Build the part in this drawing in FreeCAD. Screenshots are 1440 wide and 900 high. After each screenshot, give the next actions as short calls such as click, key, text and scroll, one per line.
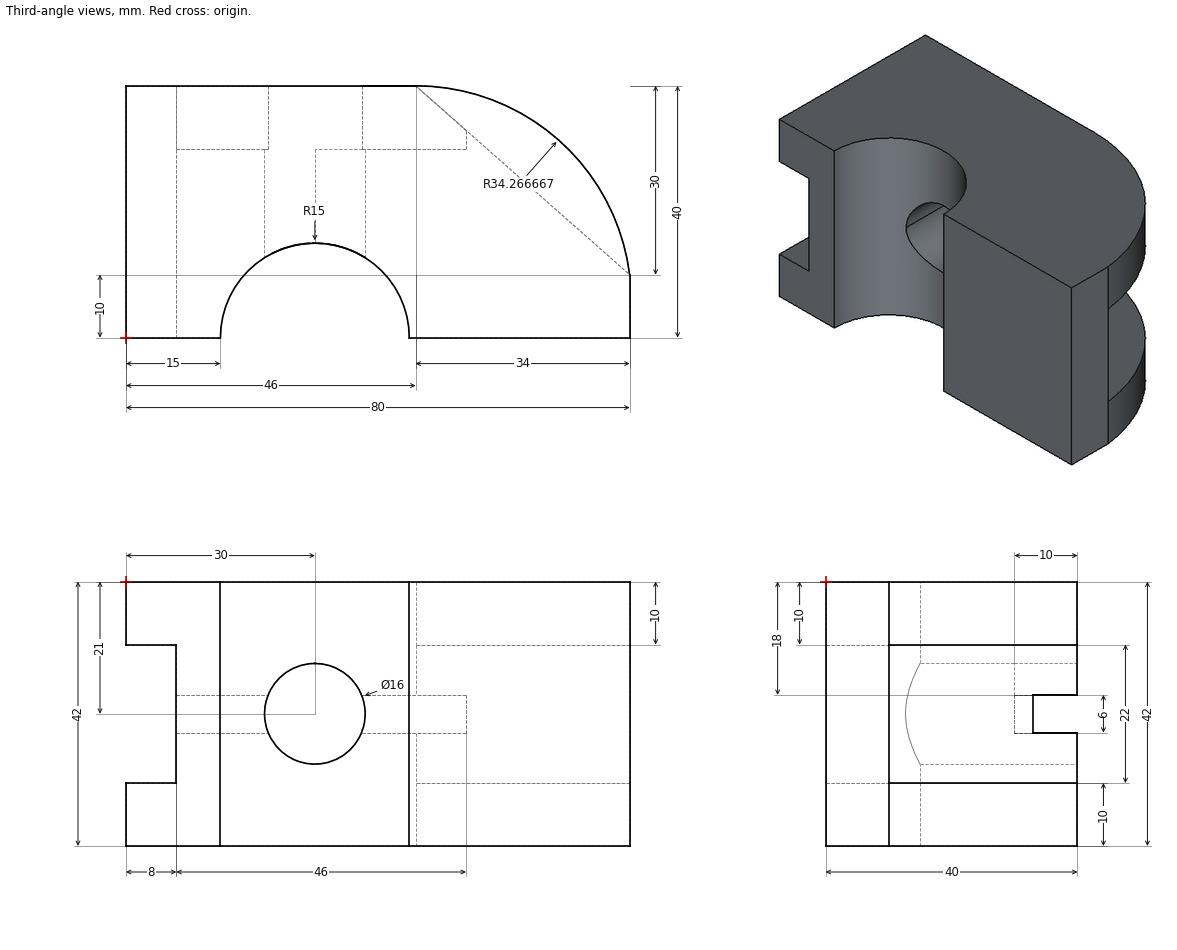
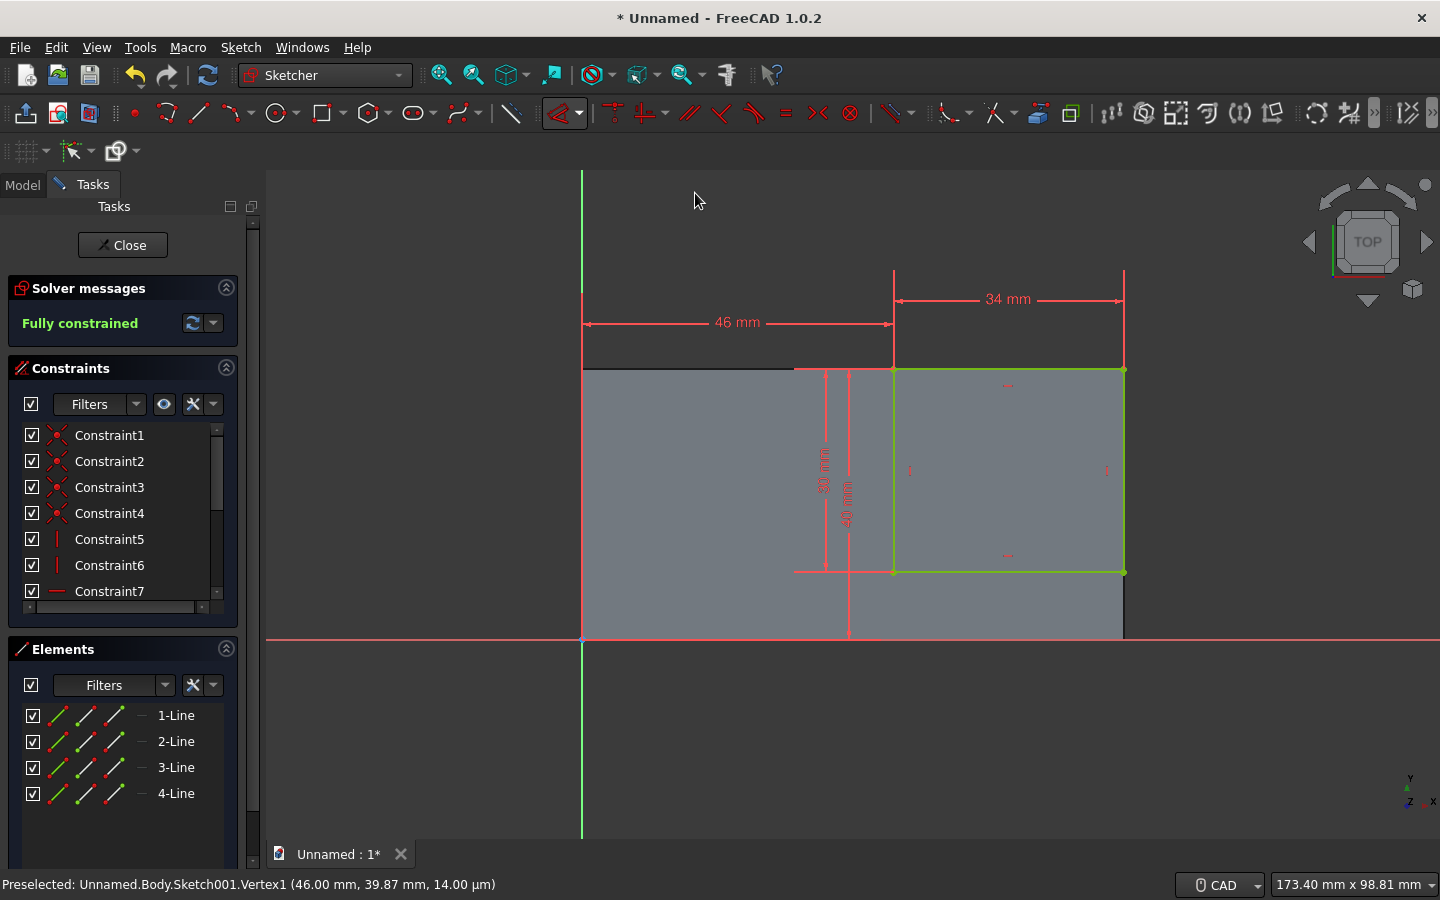
click(123, 245)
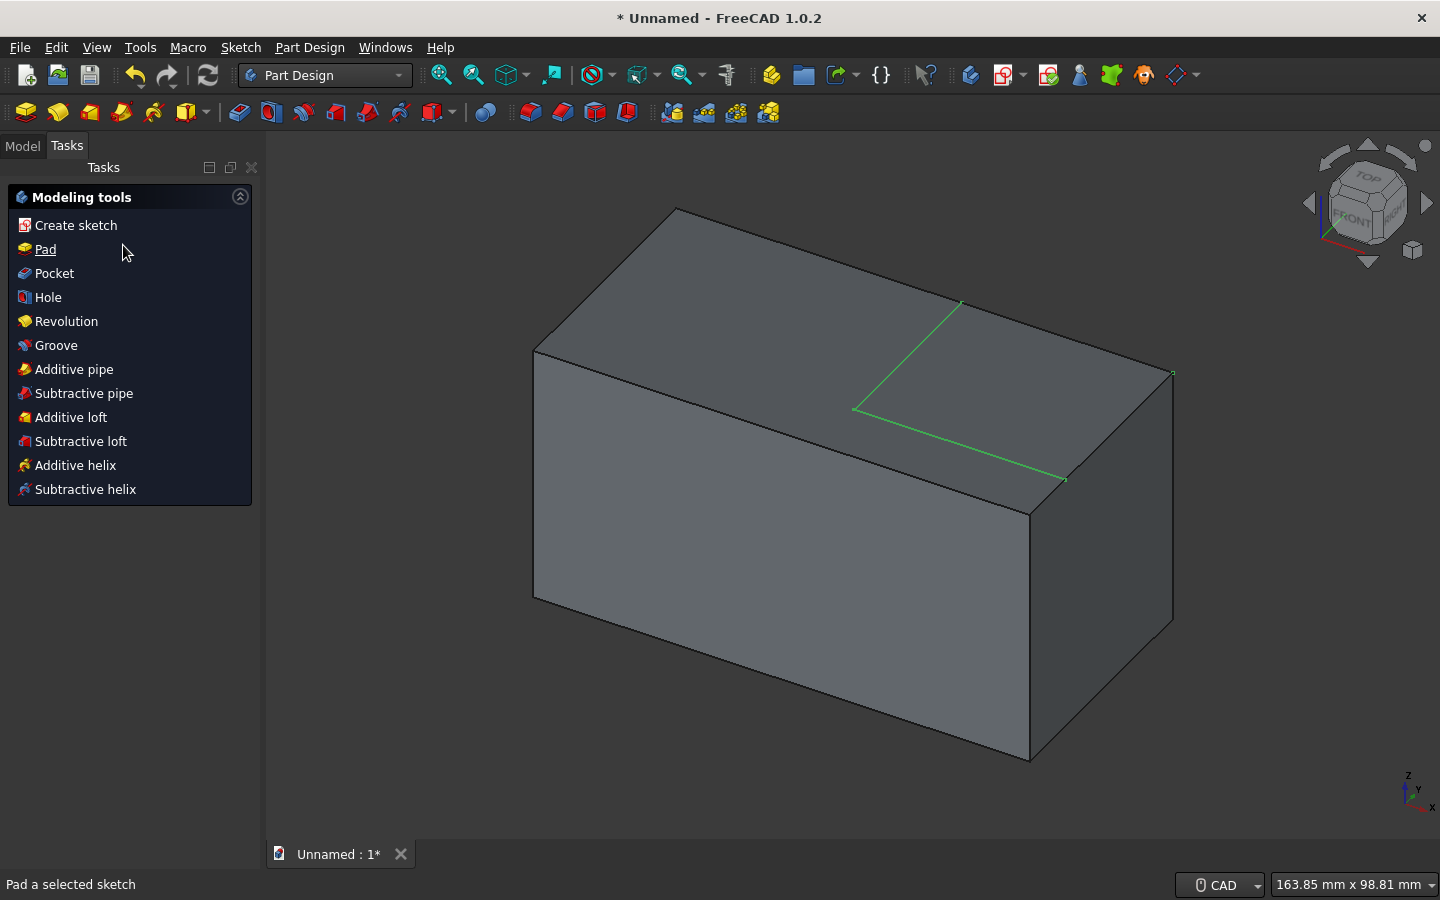
click(240, 112)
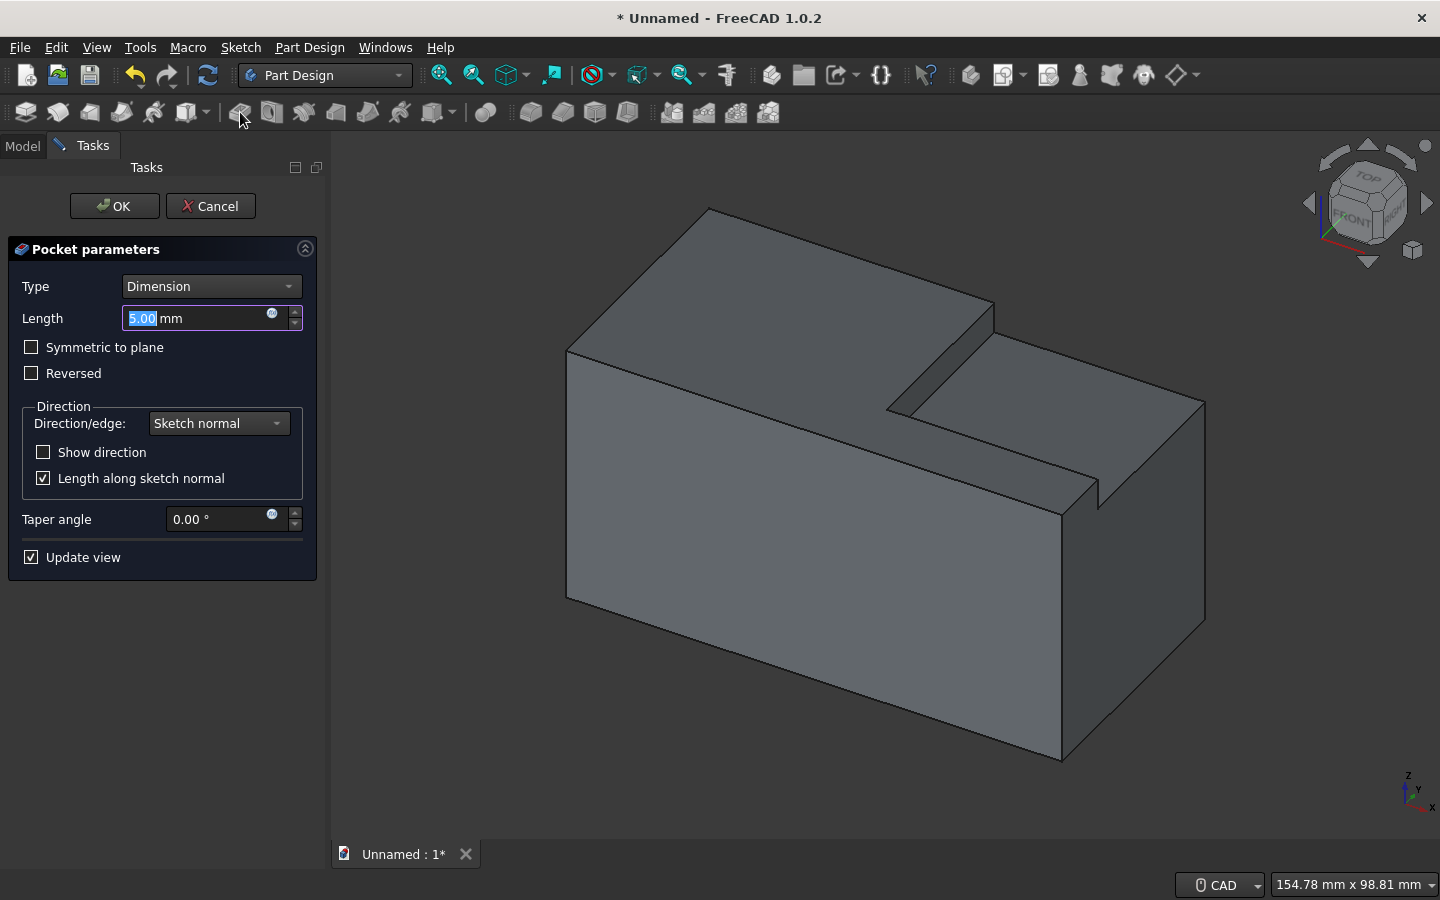
text(10)
key(Tab)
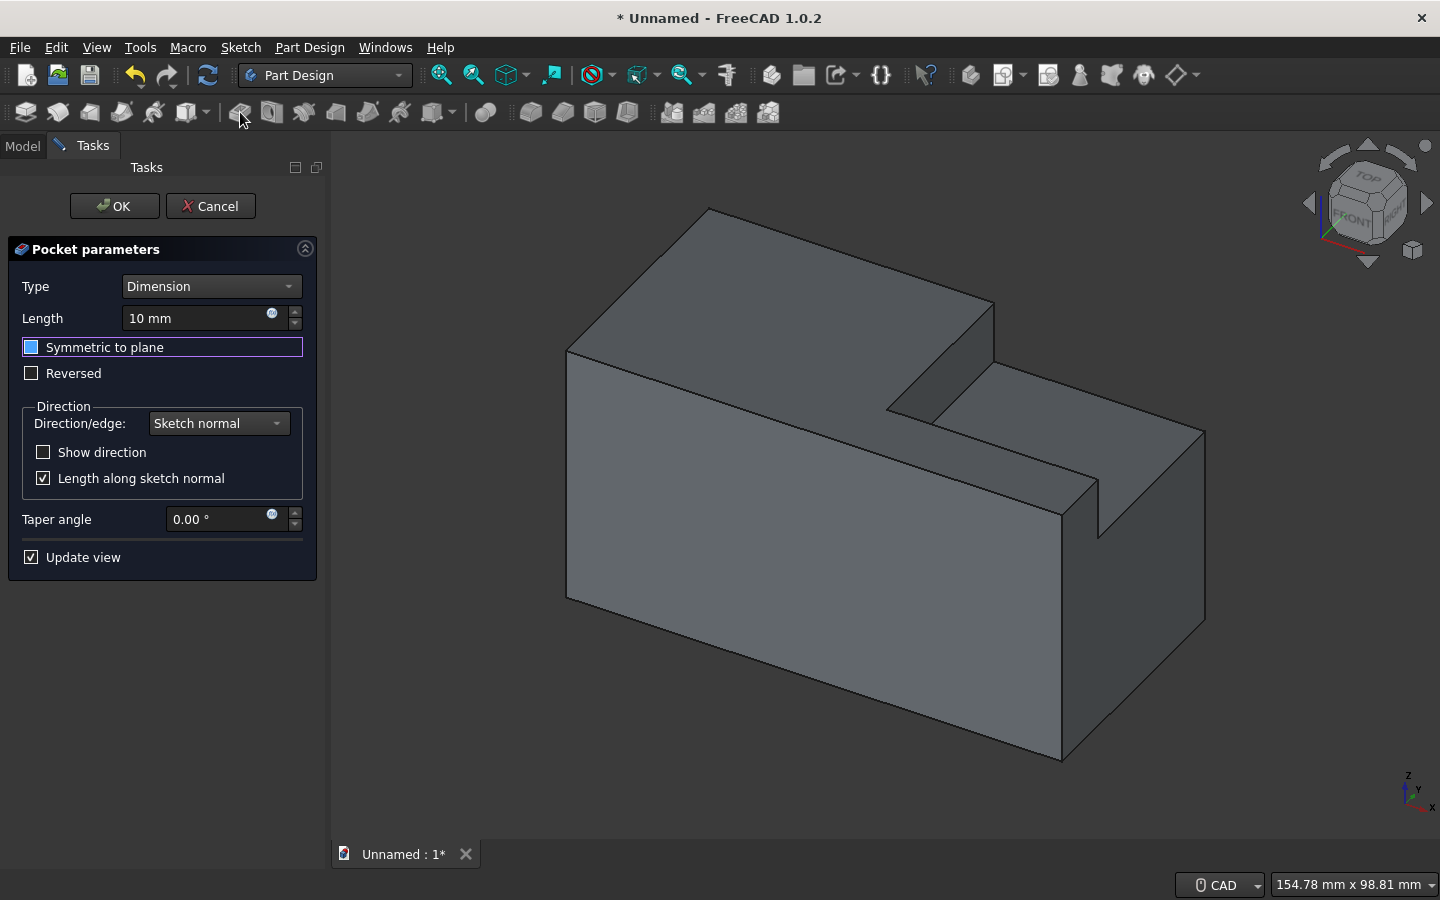
click(115, 206)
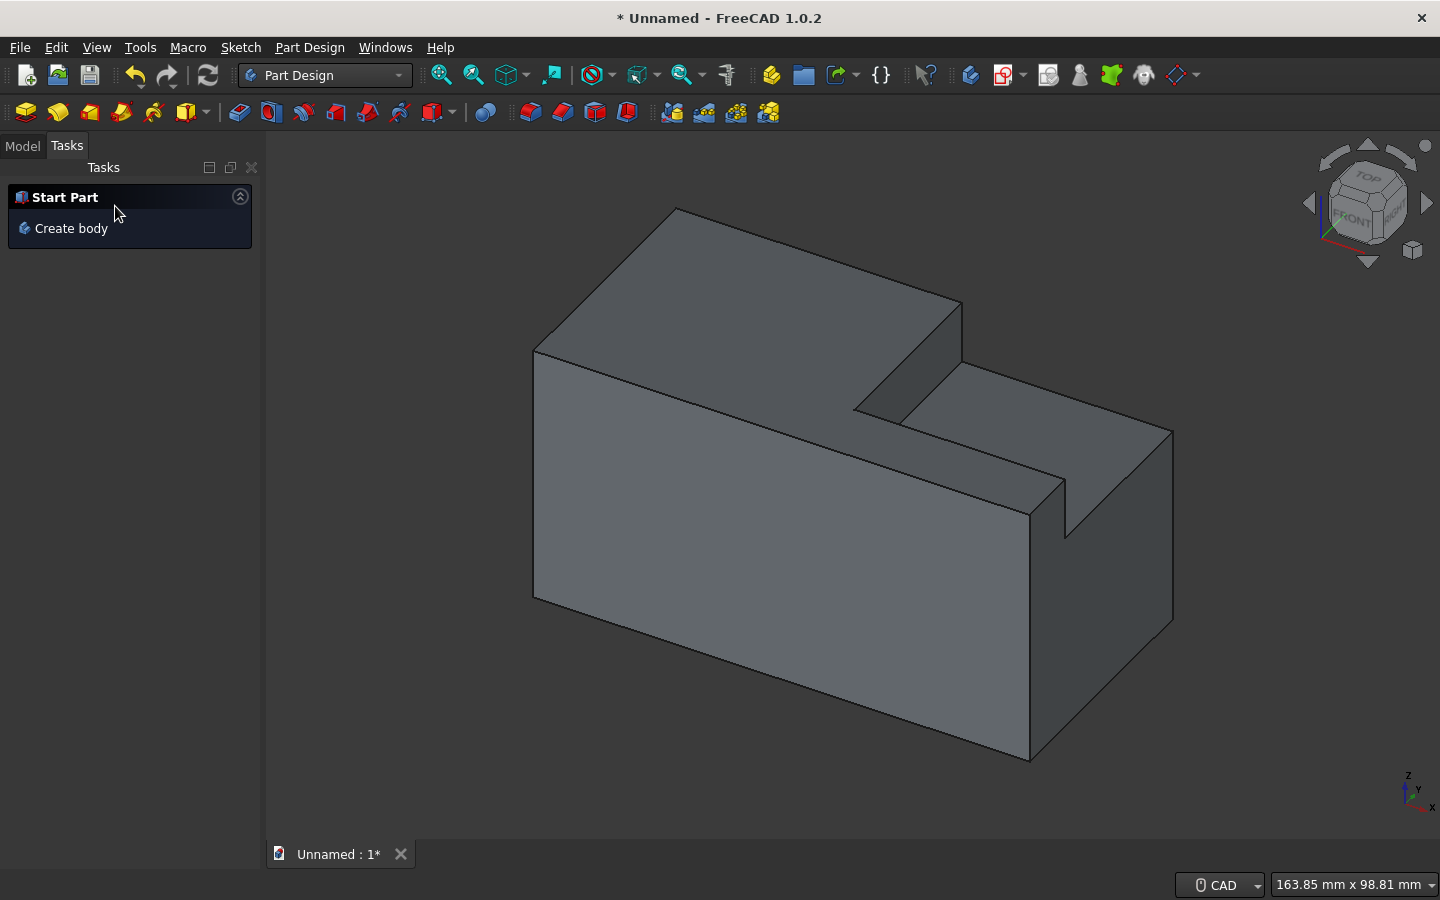
click(1014, 449)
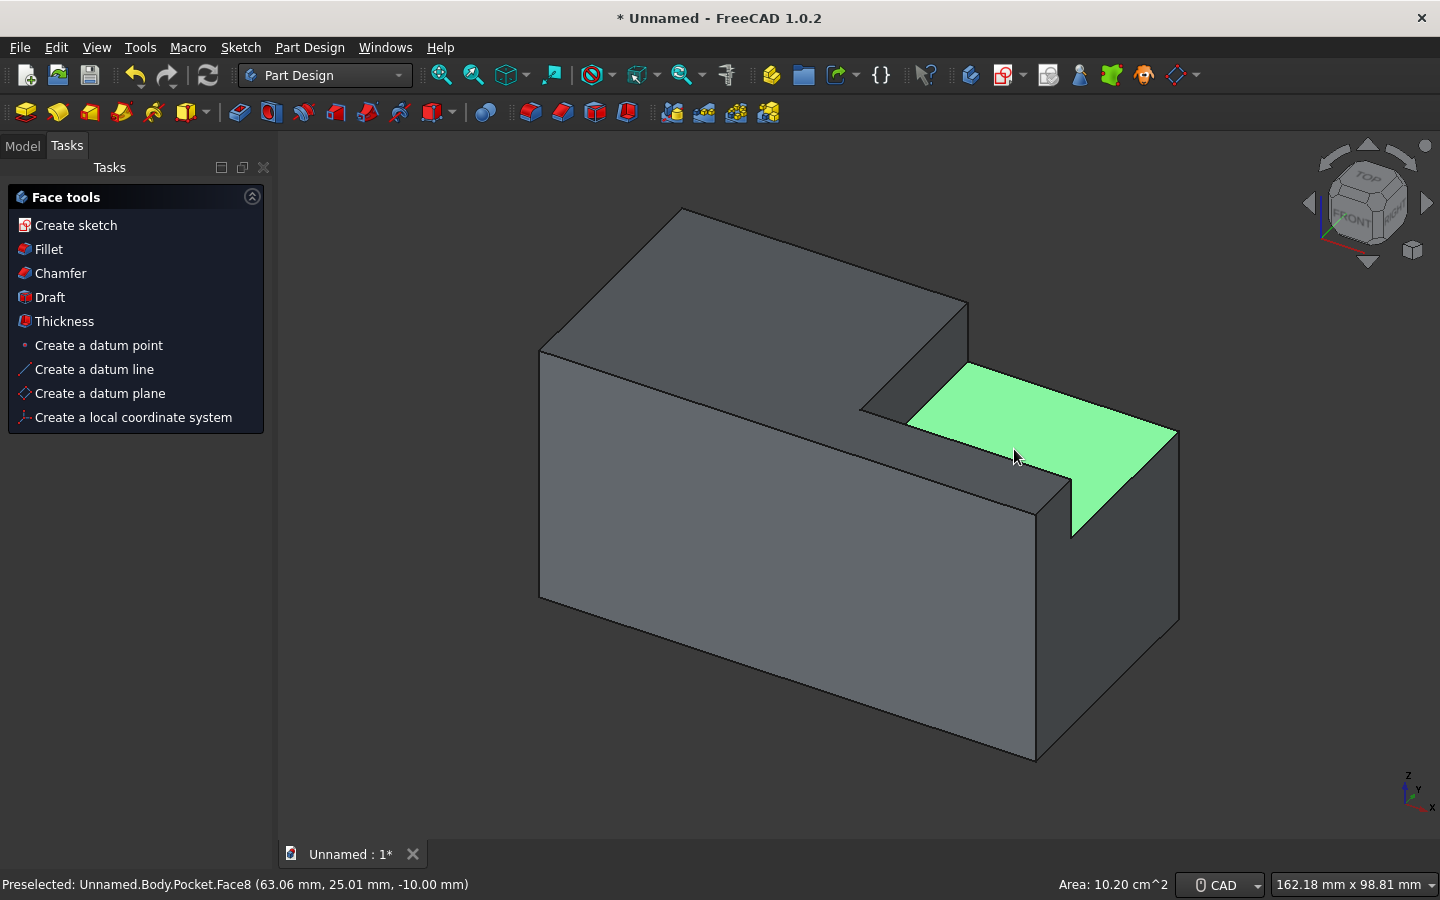
click(1004, 76)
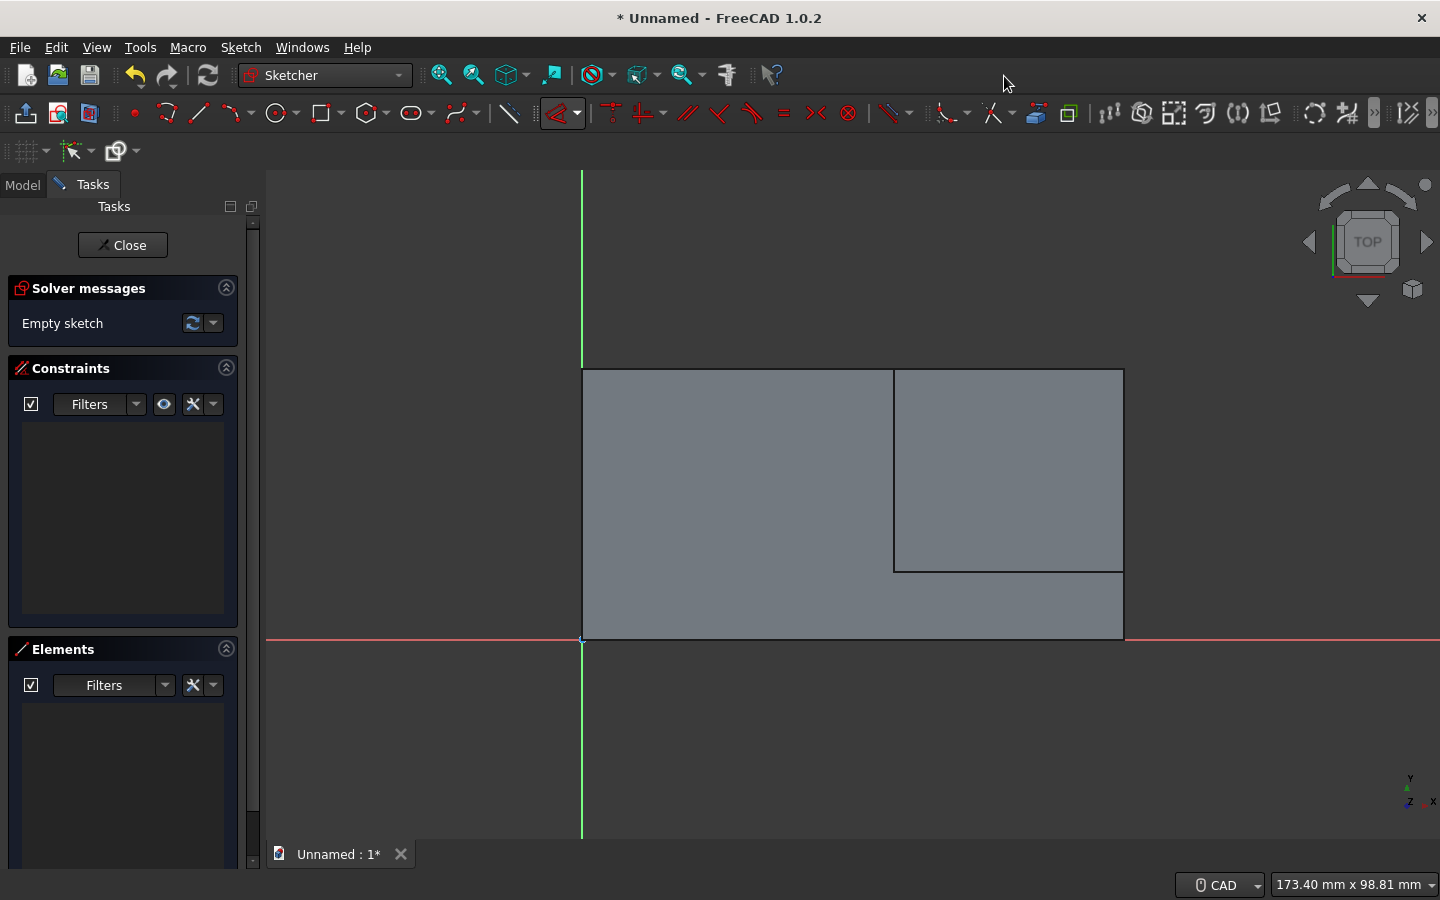
click(90, 114)